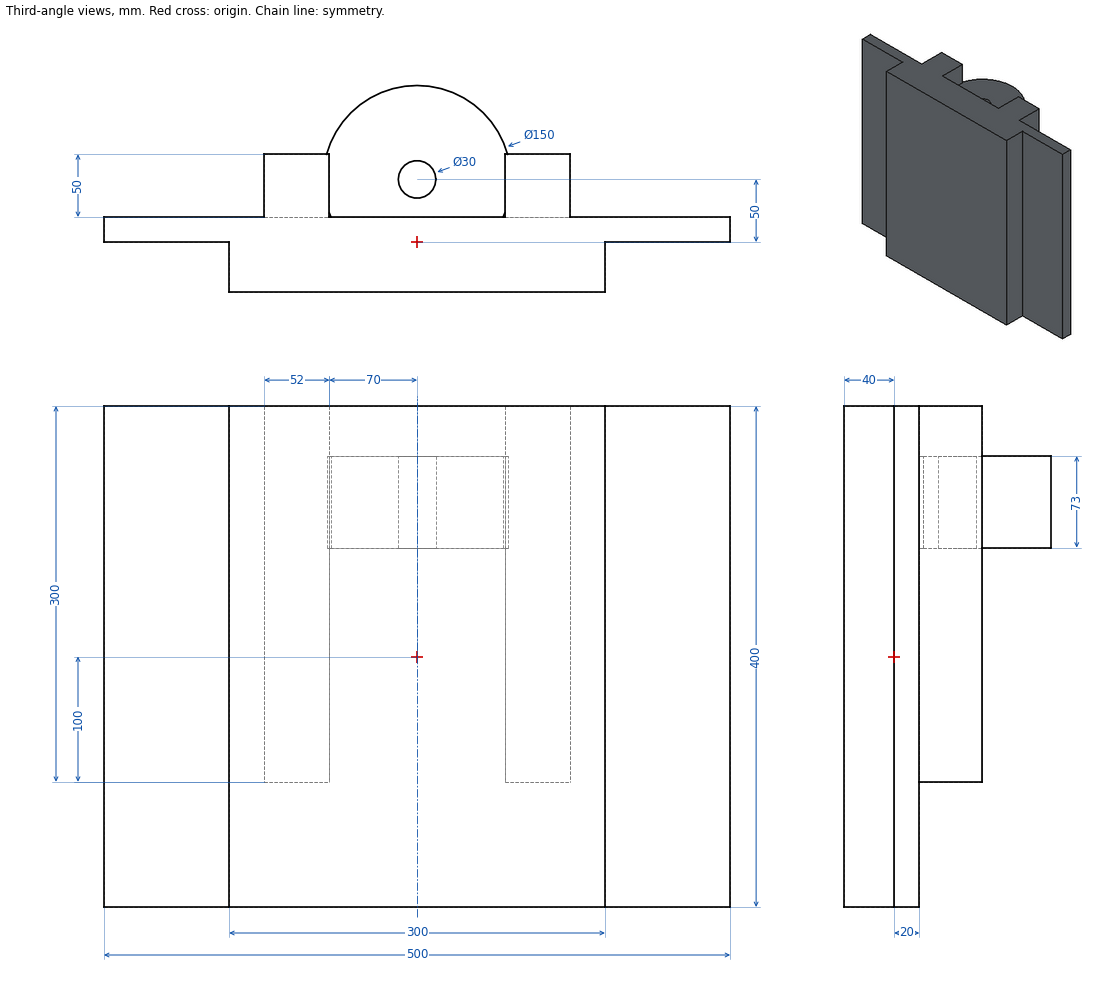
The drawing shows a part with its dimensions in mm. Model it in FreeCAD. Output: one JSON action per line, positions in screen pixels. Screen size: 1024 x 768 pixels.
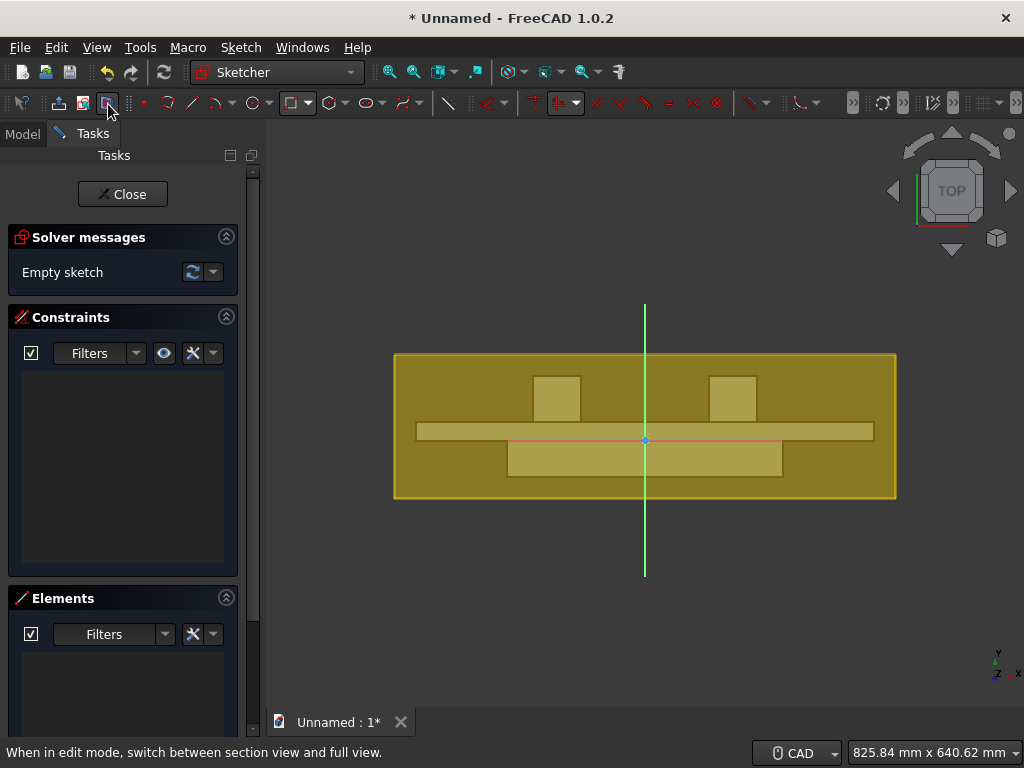
{"action": "scroll", "coordinate": [685, 384], "scroll_direction": "up", "scroll_amount": 5}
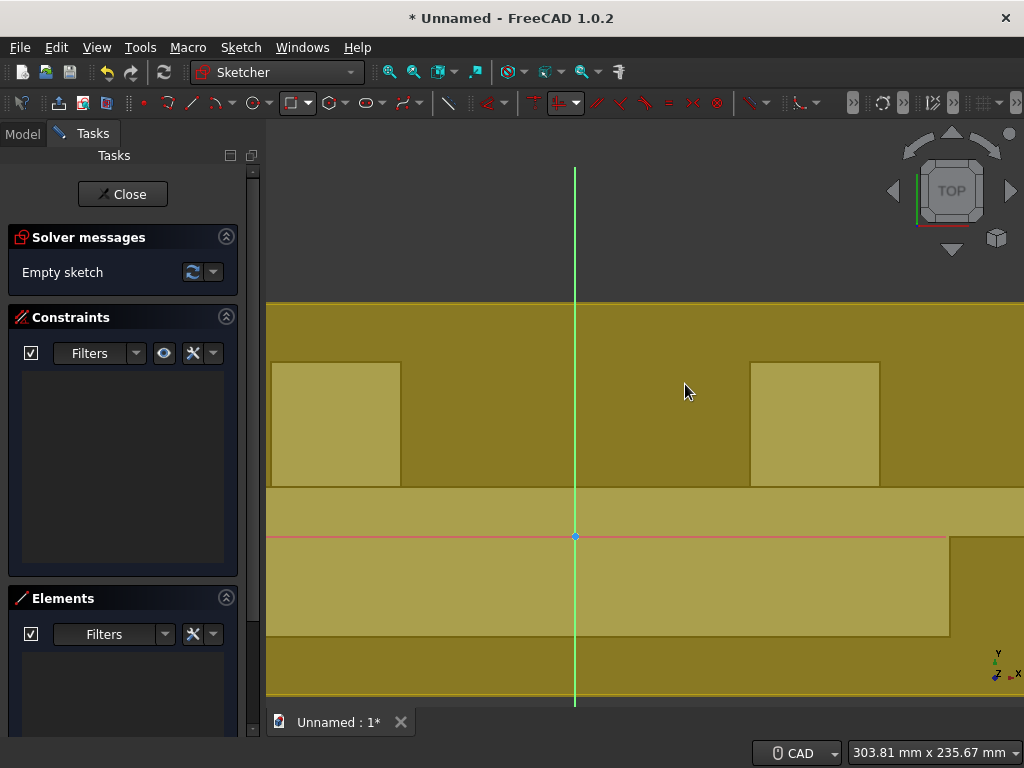
{"action": "left_click", "coordinate": [254, 104]}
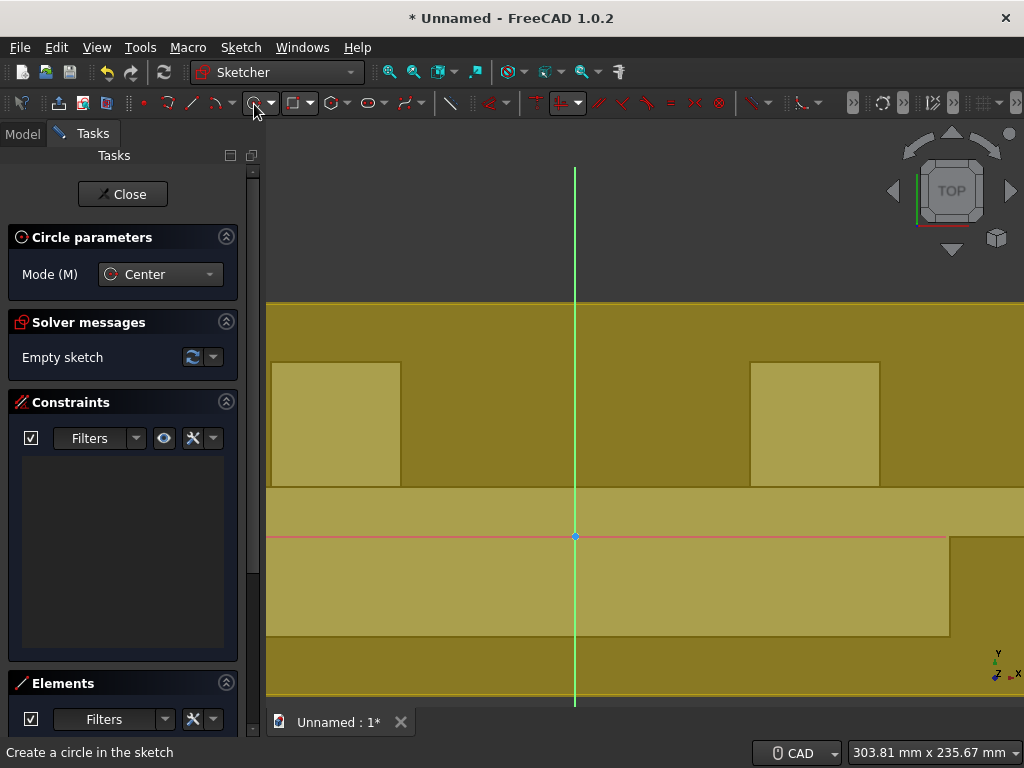
{"action": "left_click", "coordinate": [575, 412]}
{"action": "left_click", "coordinate": [708, 280]}
{"action": "key", "text": "Escape"}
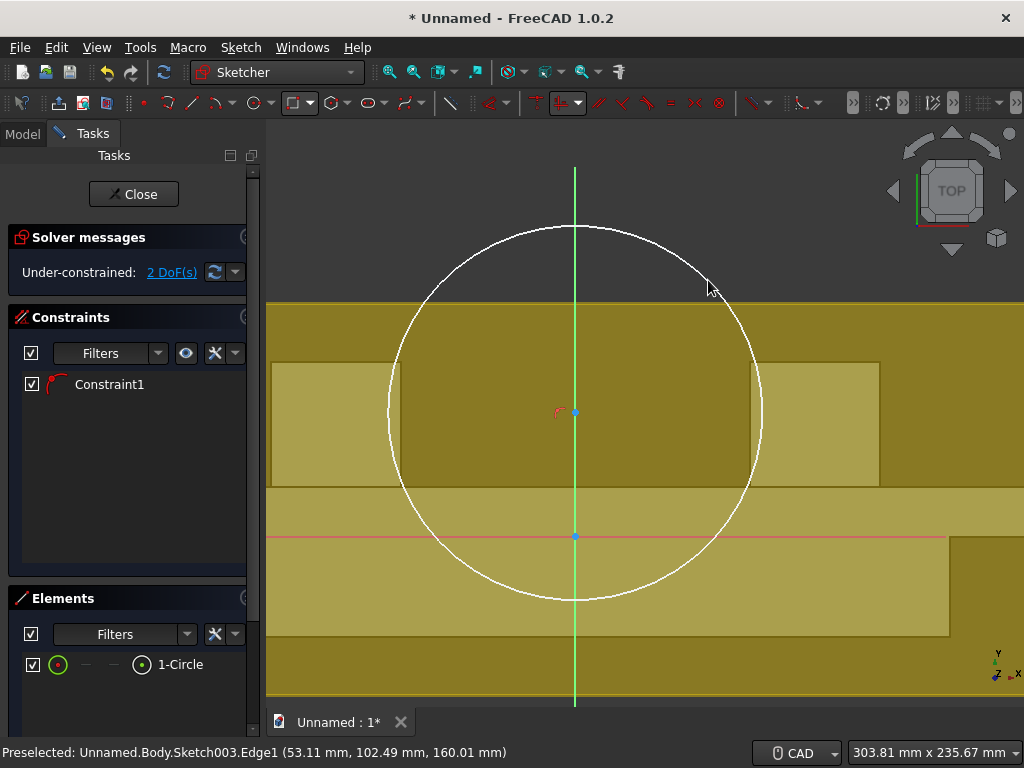
{"action": "left_click", "coordinate": [490, 104]}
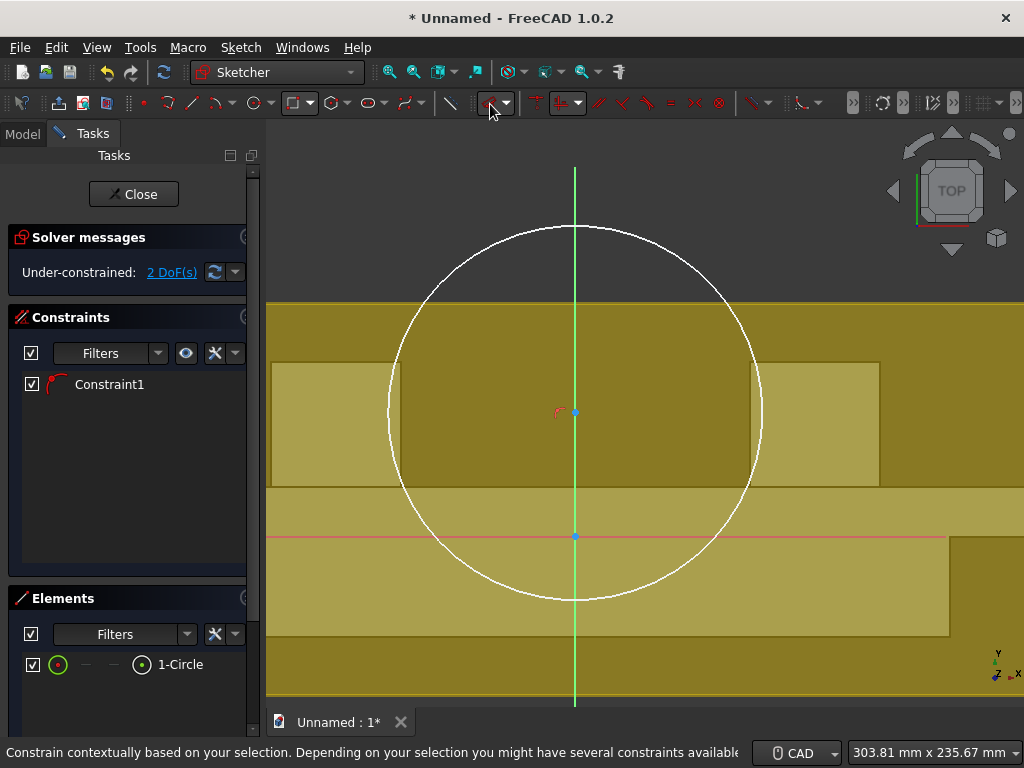
{"action": "left_click", "coordinate": [707, 280]}
{"action": "left_click", "coordinate": [730, 257]}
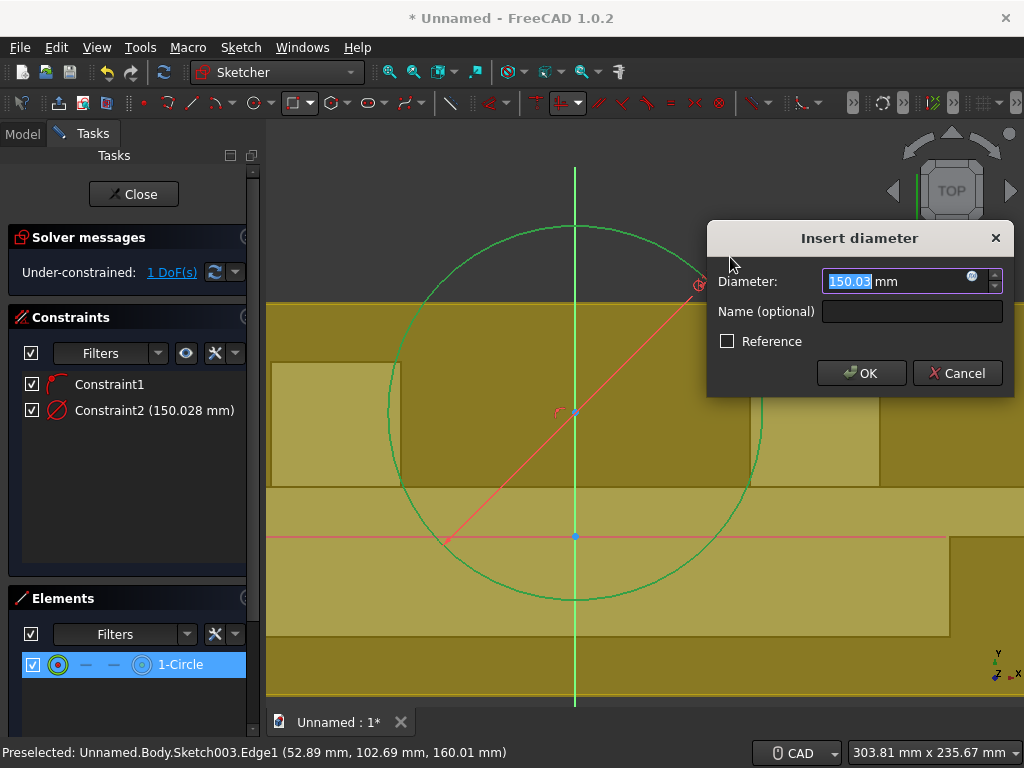
{"action": "type", "text": "150"}
{"action": "key", "text": "Return"}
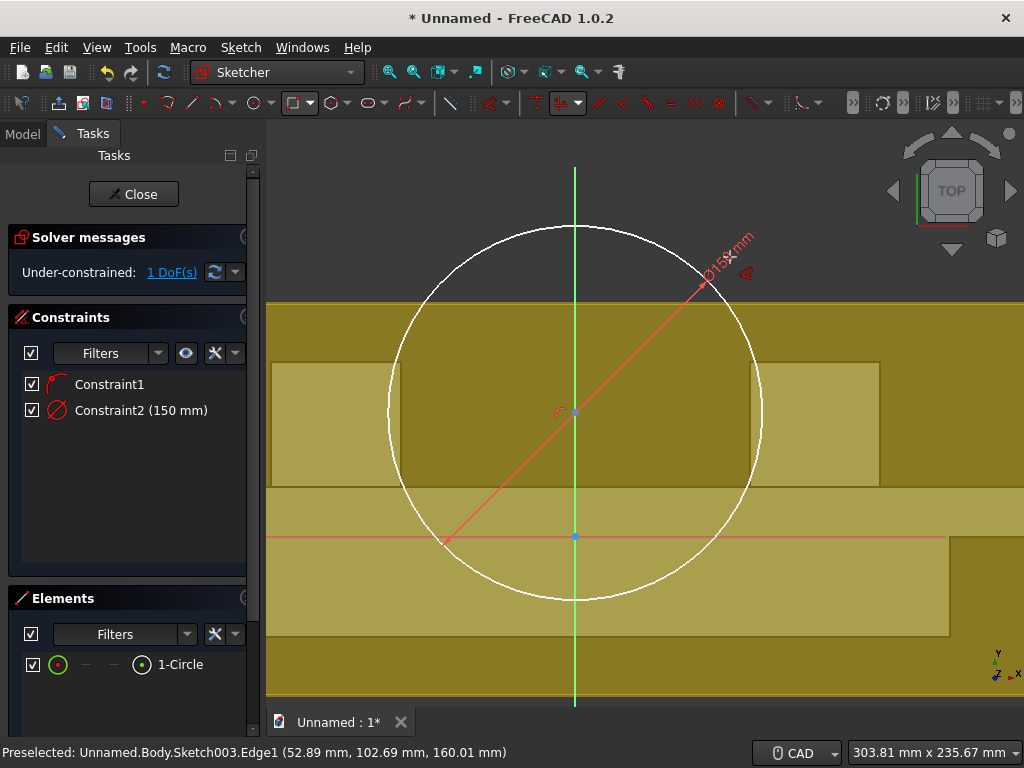
{"action": "left_click", "coordinate": [575, 413]}
{"action": "left_click", "coordinate": [609, 475]}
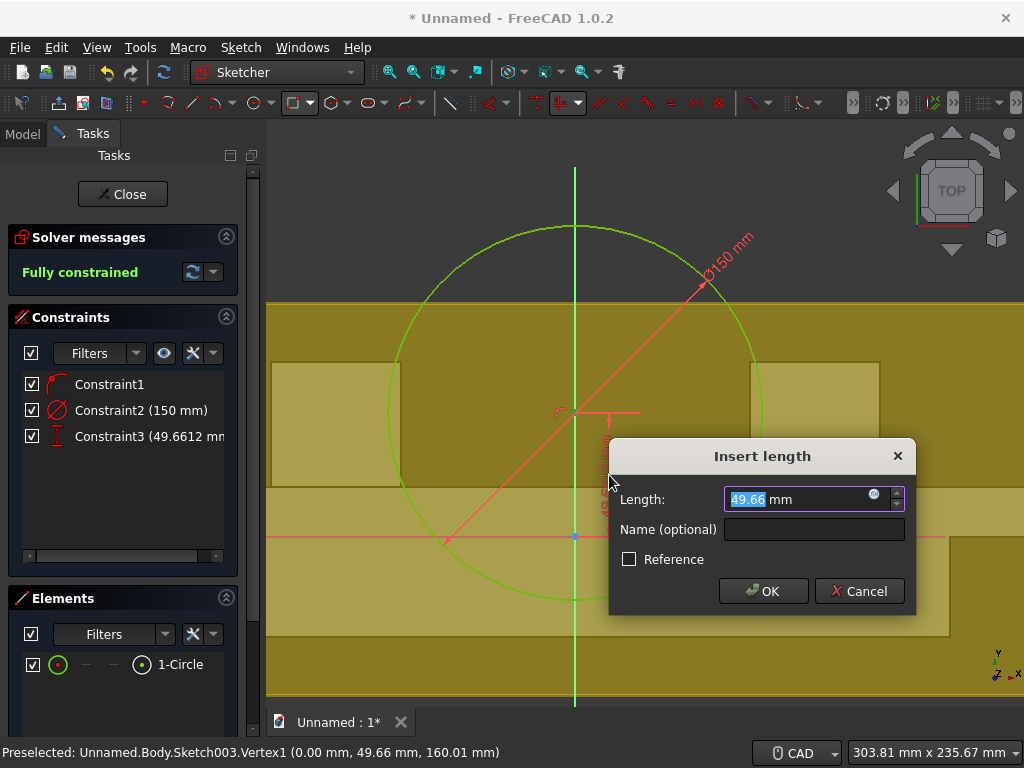
{"action": "type", "text": "50"}
{"action": "key", "text": "Return"}
{"action": "key", "text": "Escape"}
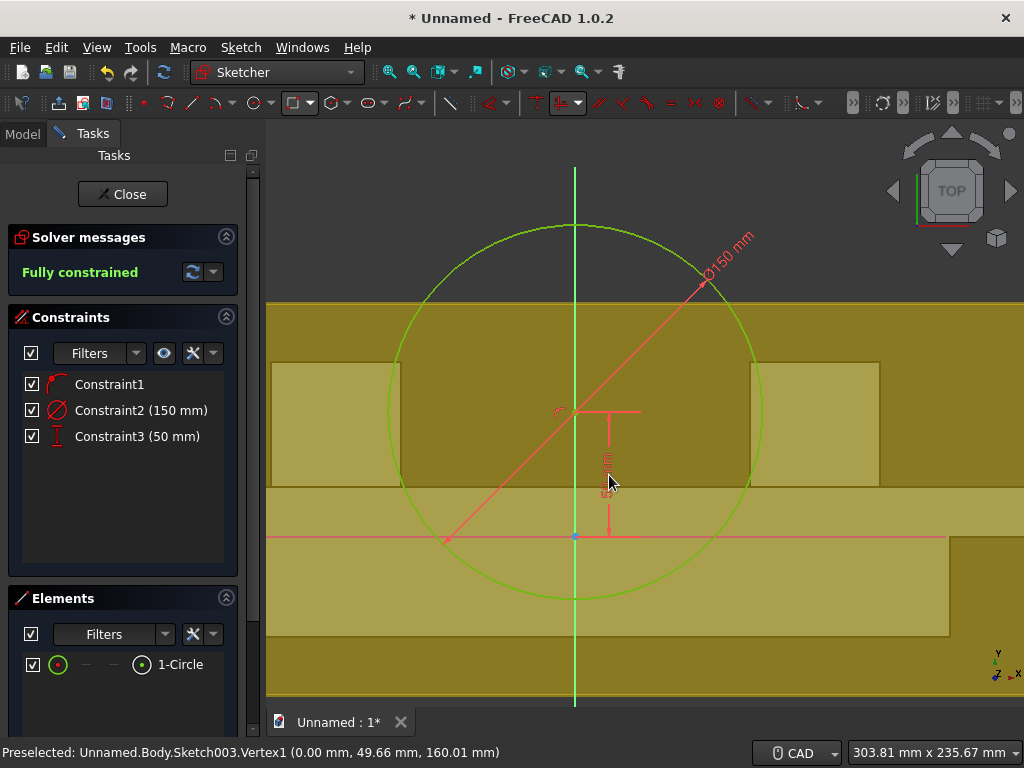
{"action": "left_click", "coordinate": [123, 194]}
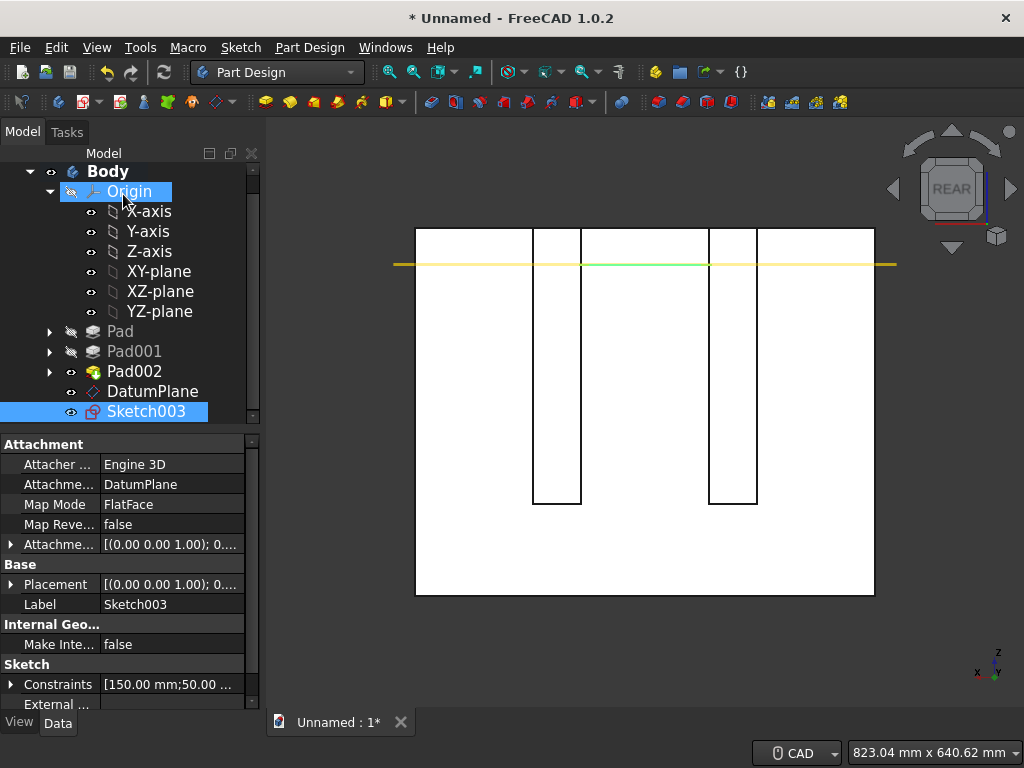
{"action": "left_click", "coordinate": [266, 102]}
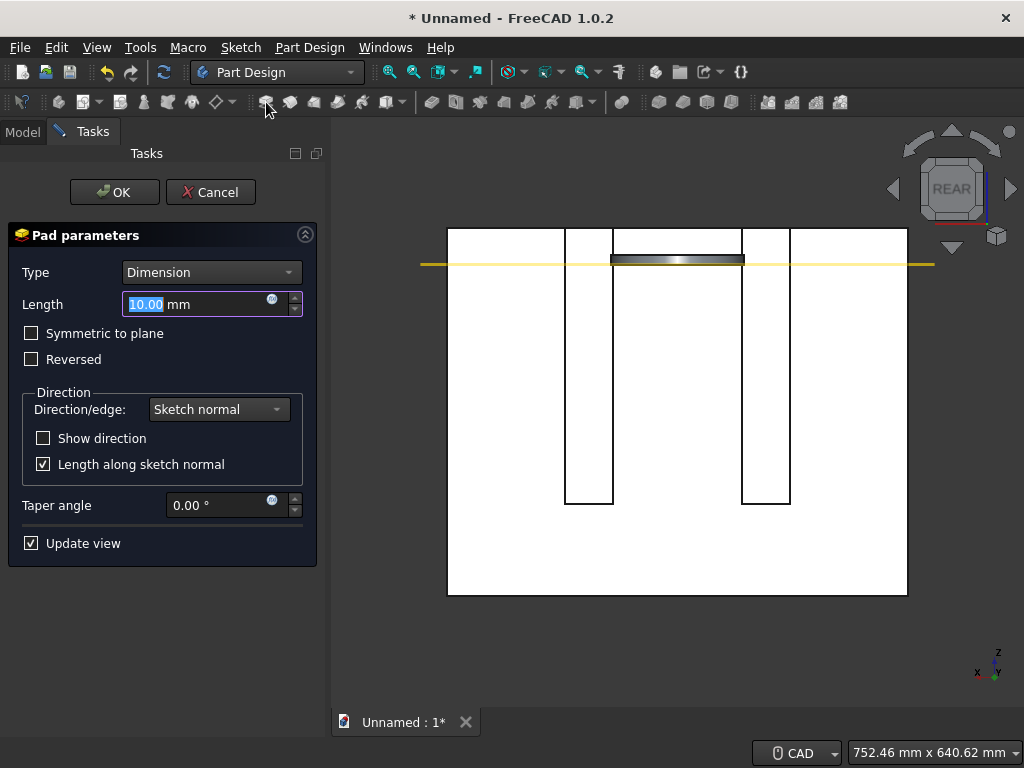
{"action": "type", "text": "73"}
{"action": "key", "text": "Tab"}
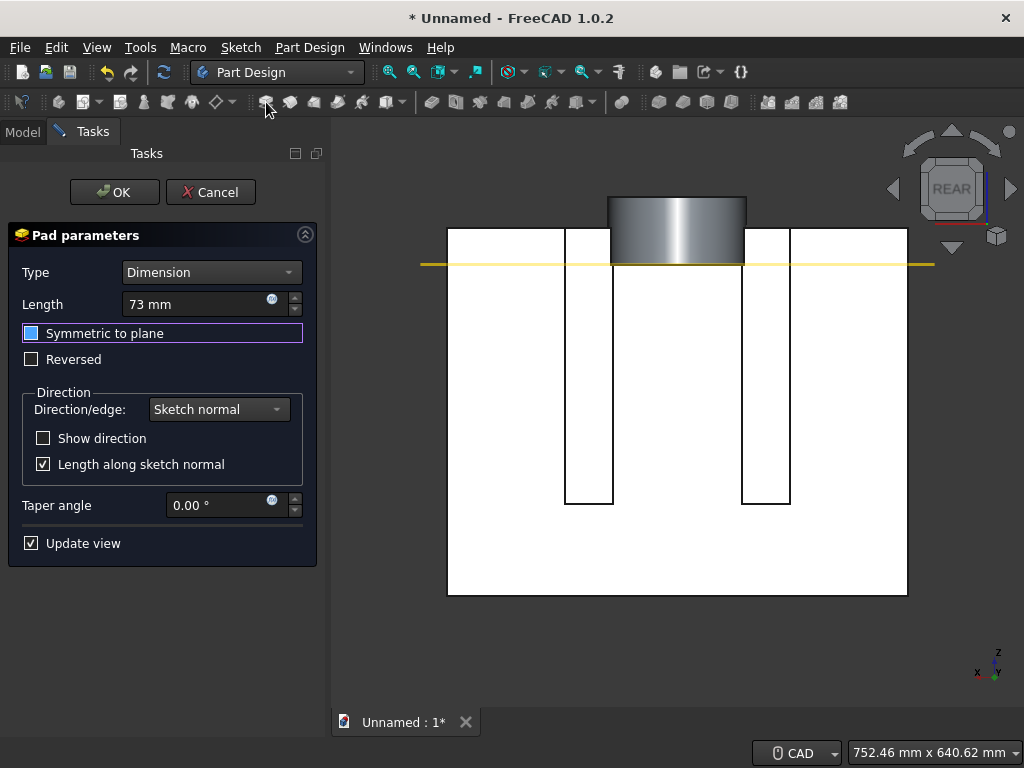
{"action": "left_click", "coordinate": [30, 359]}